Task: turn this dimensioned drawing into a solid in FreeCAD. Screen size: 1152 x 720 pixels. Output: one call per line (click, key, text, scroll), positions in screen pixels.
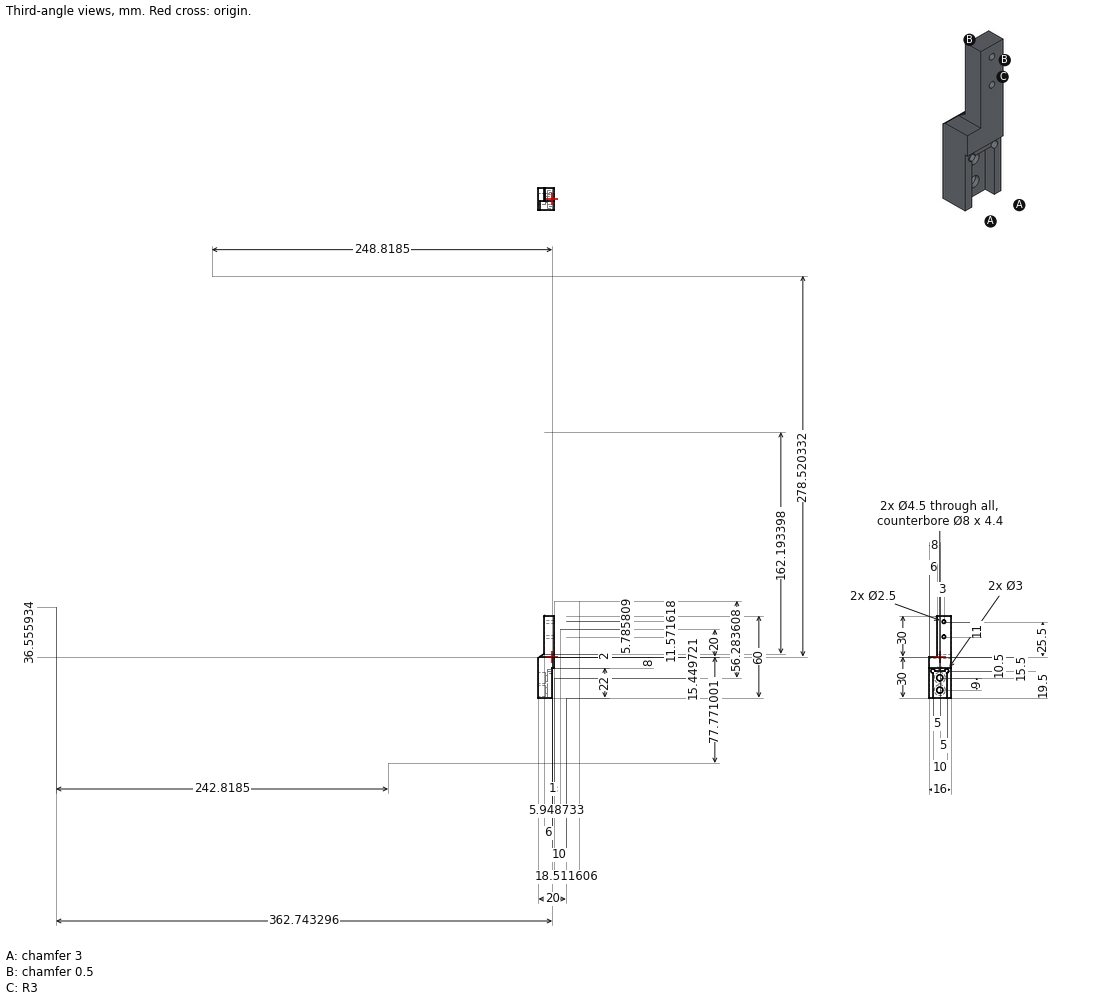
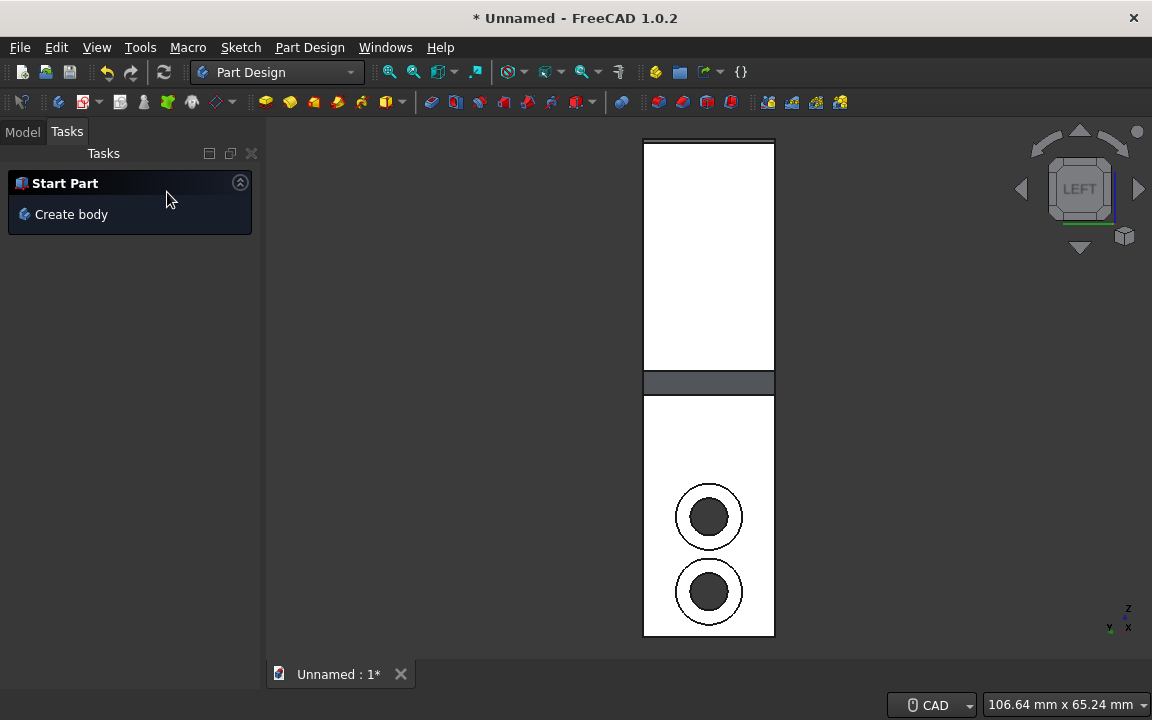
key(0)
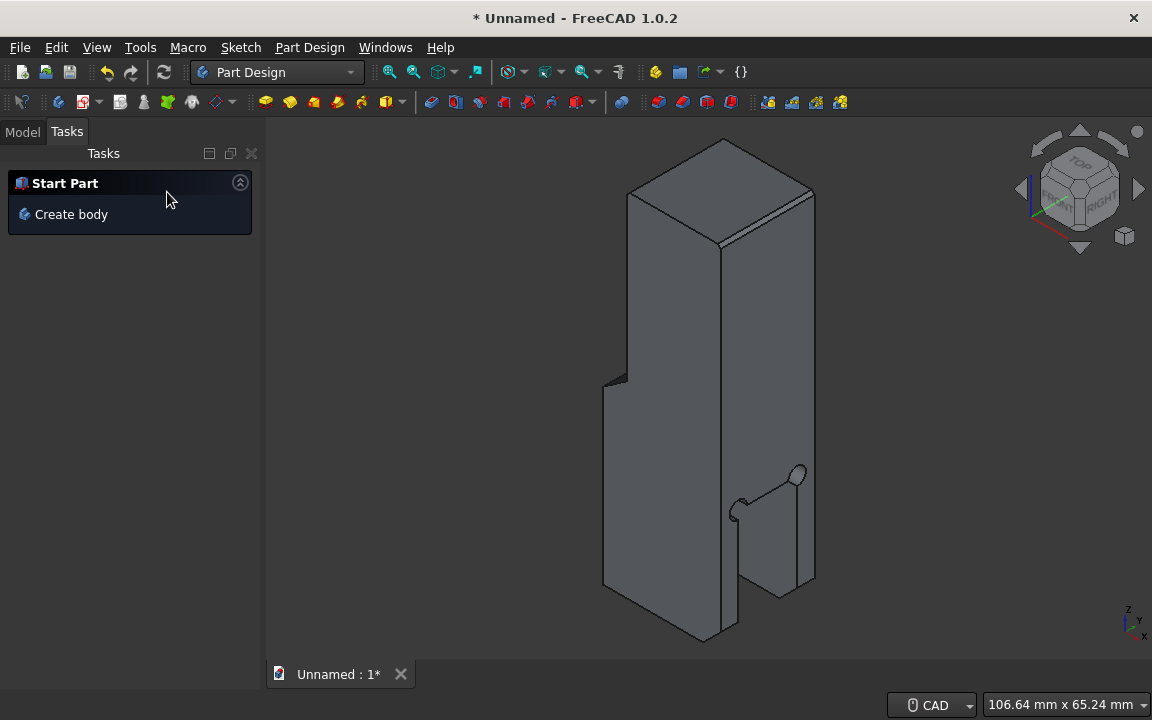
click(662, 472)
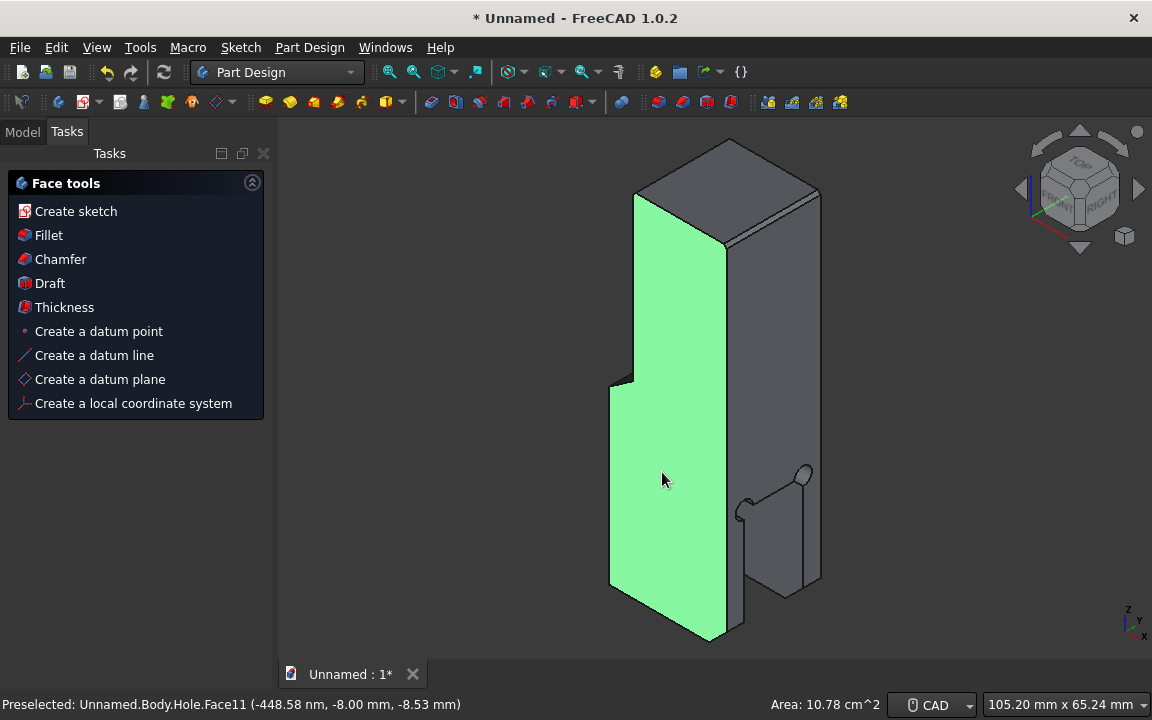
click(84, 102)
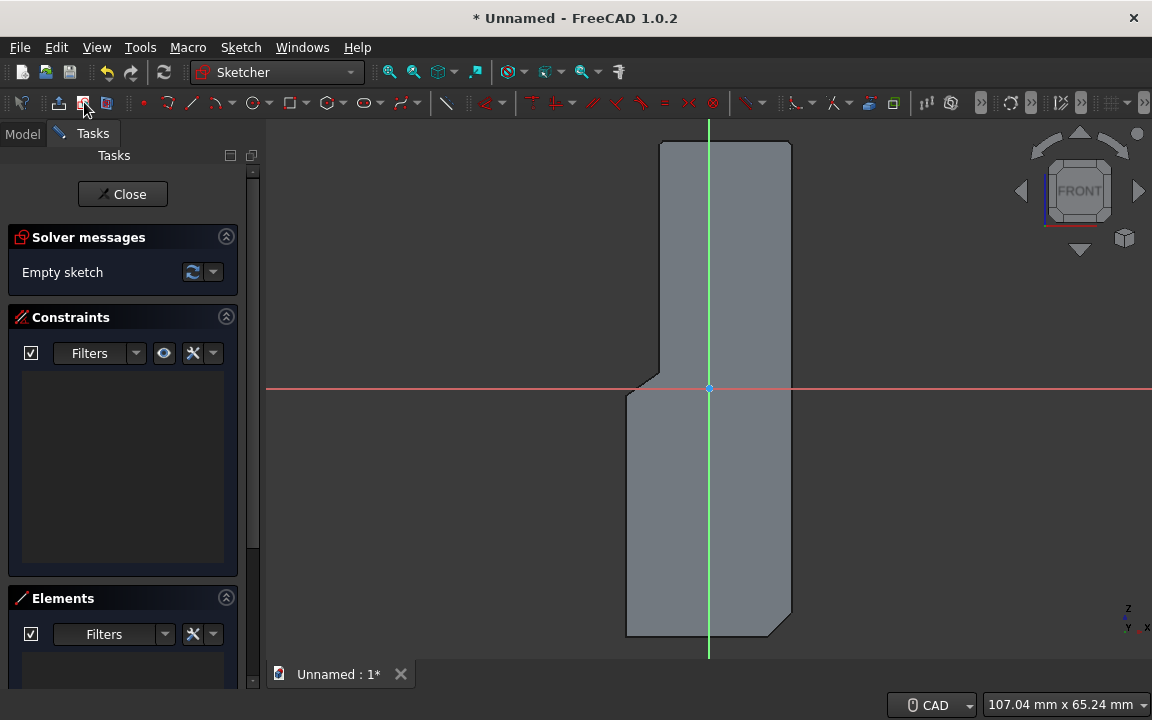
scroll(294, 147, down, 1)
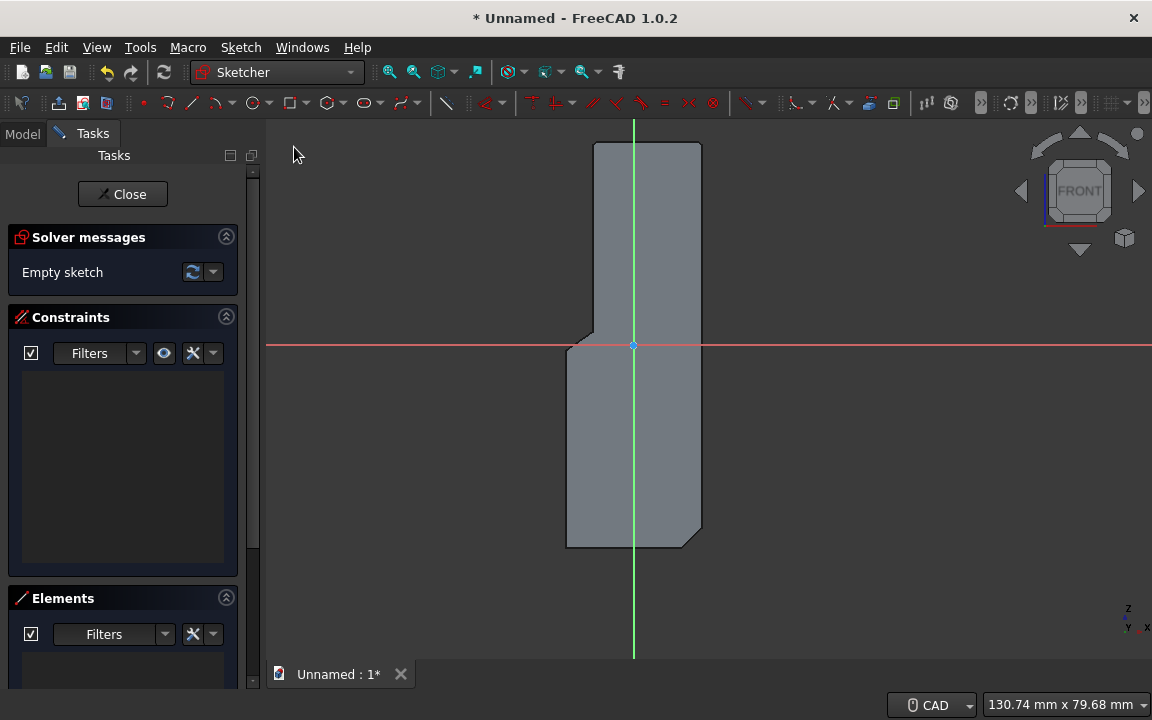
scroll(701, 517, up, 3)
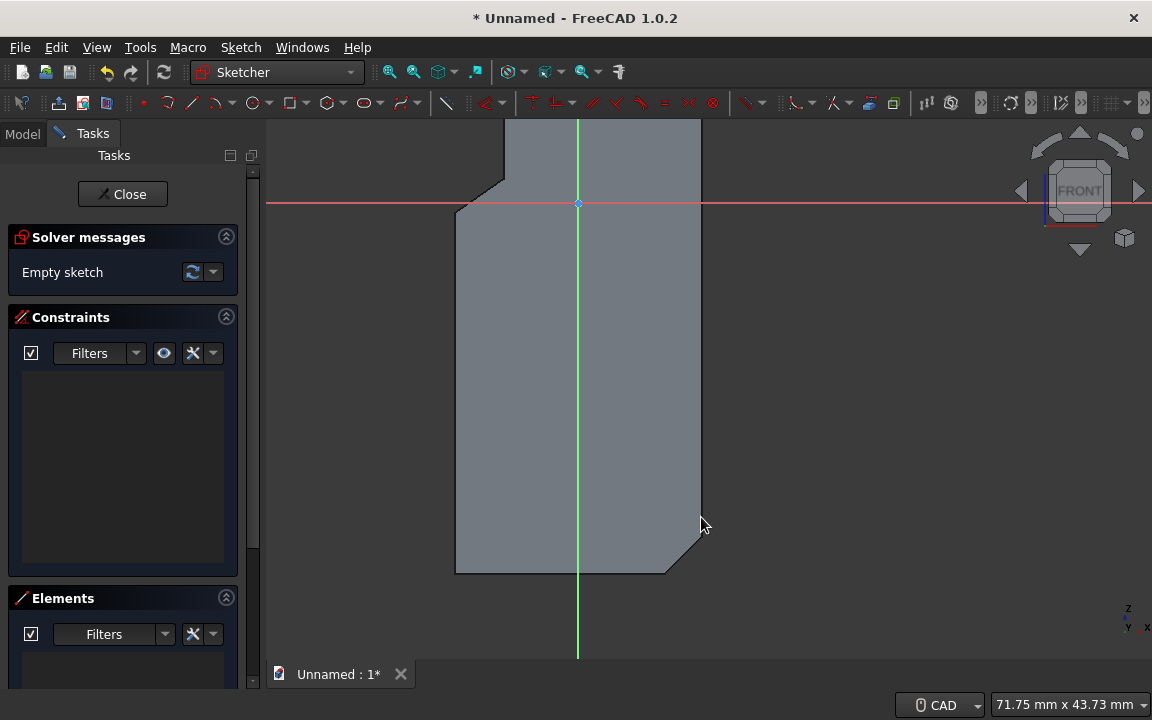
click(290, 104)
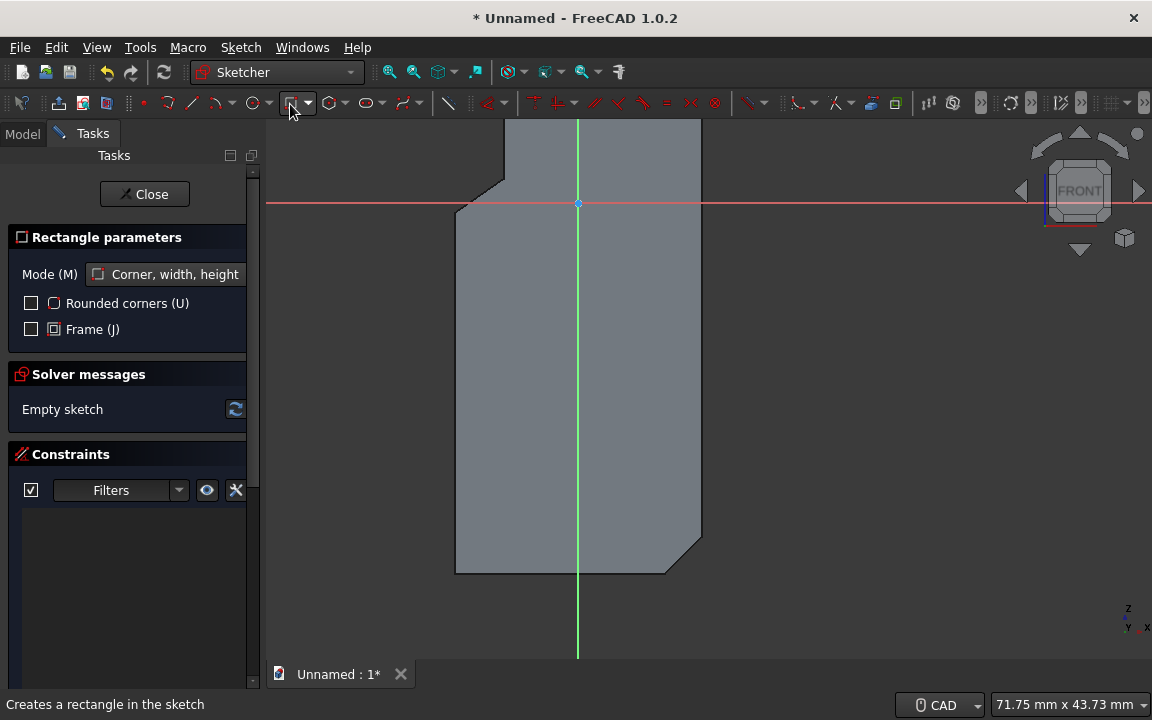
click(578, 302)
click(702, 574)
key(Escape)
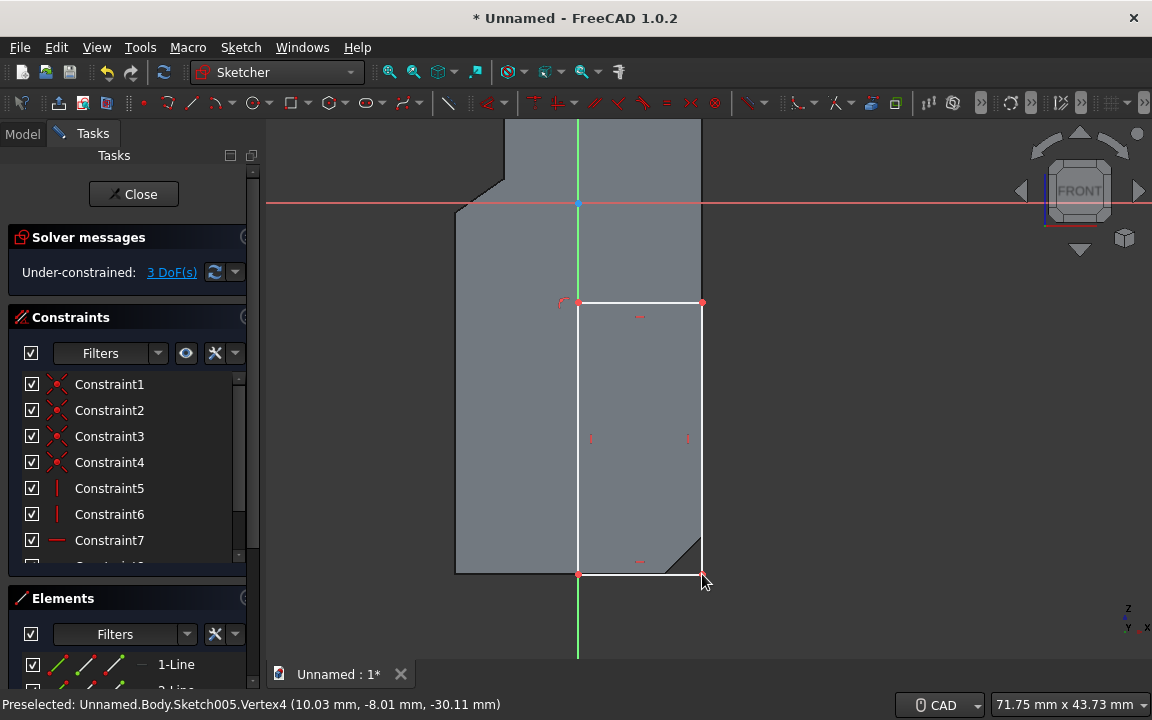
click(488, 104)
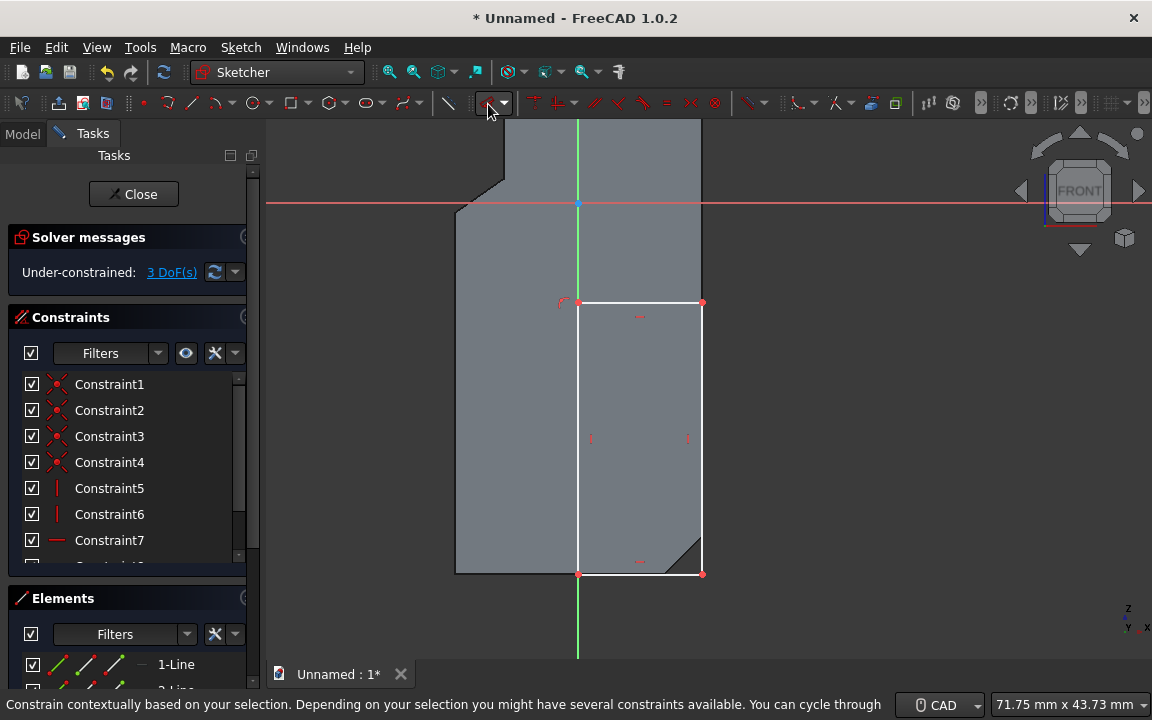
click(578, 385)
click(544, 439)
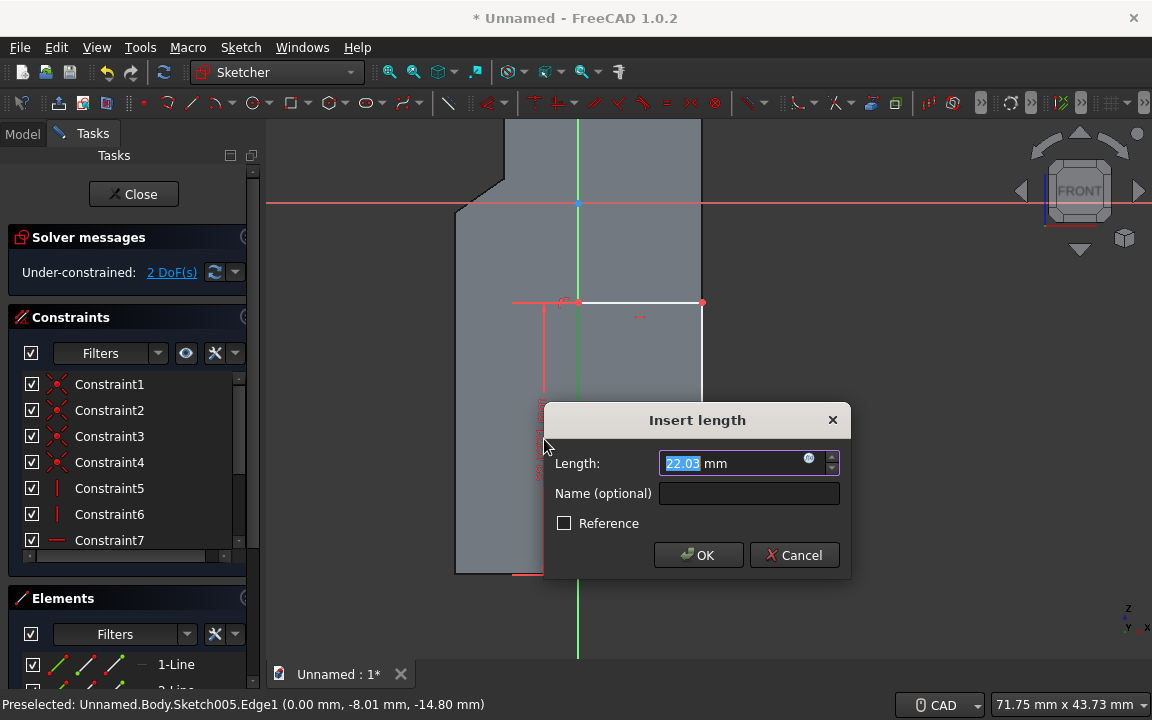
text(22)
key(Return)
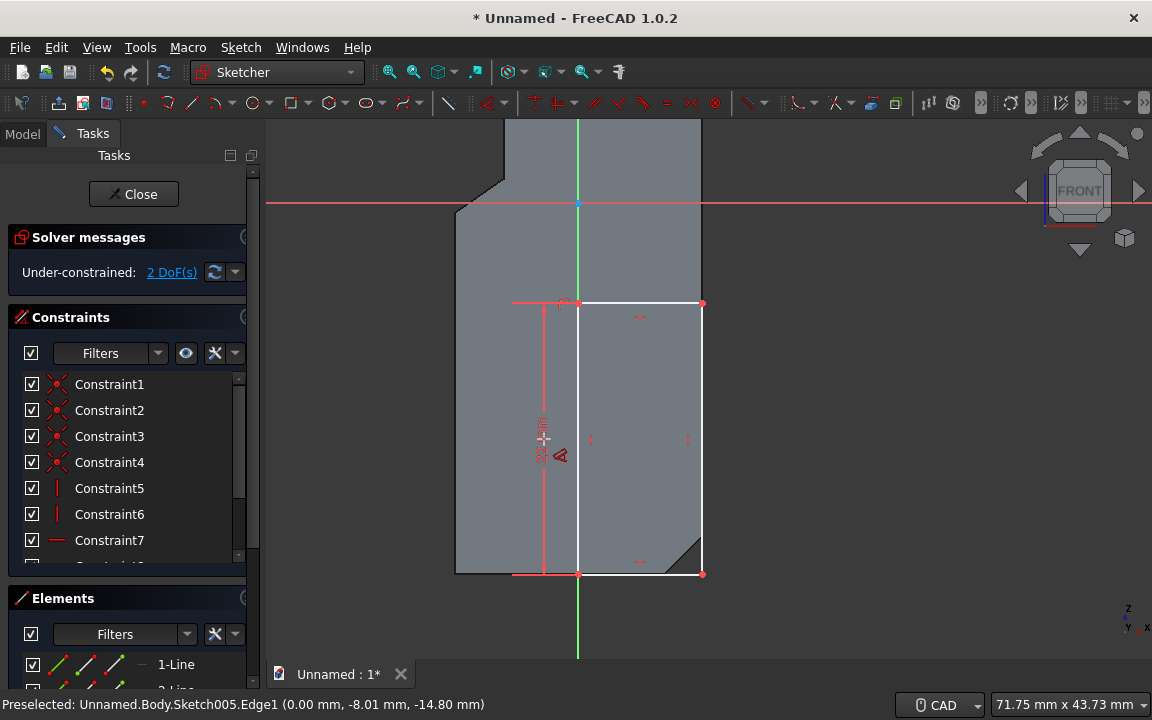
click(615, 575)
click(640, 609)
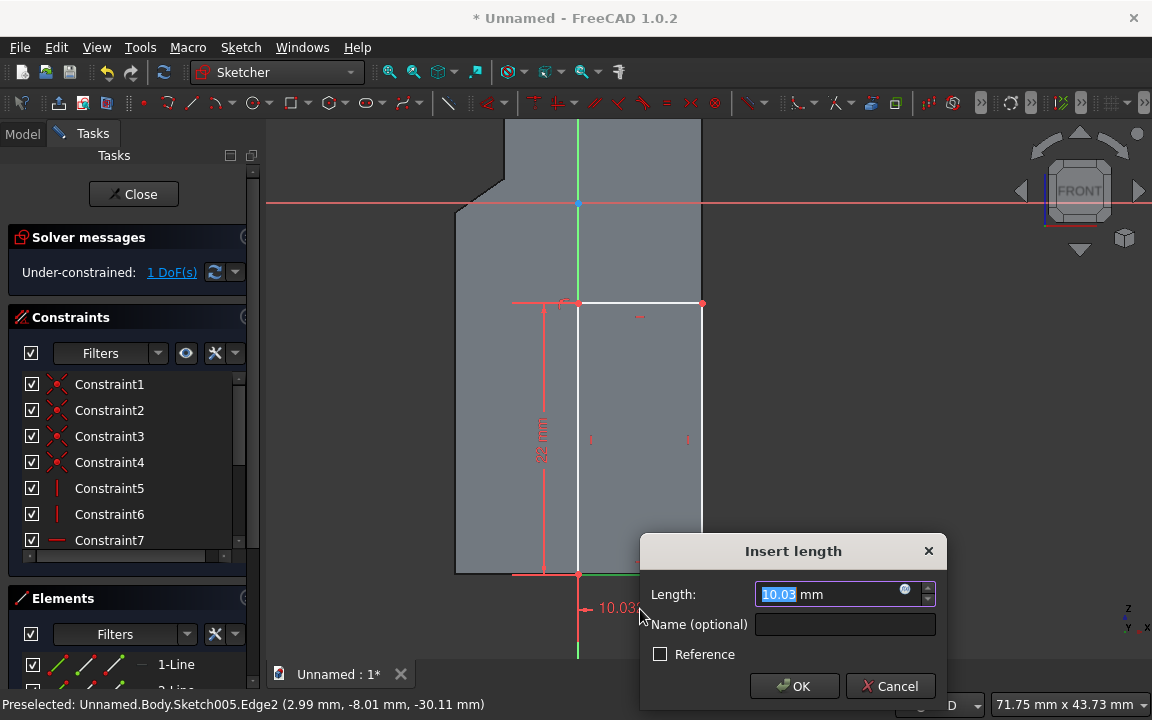
text(10)
key(Return)